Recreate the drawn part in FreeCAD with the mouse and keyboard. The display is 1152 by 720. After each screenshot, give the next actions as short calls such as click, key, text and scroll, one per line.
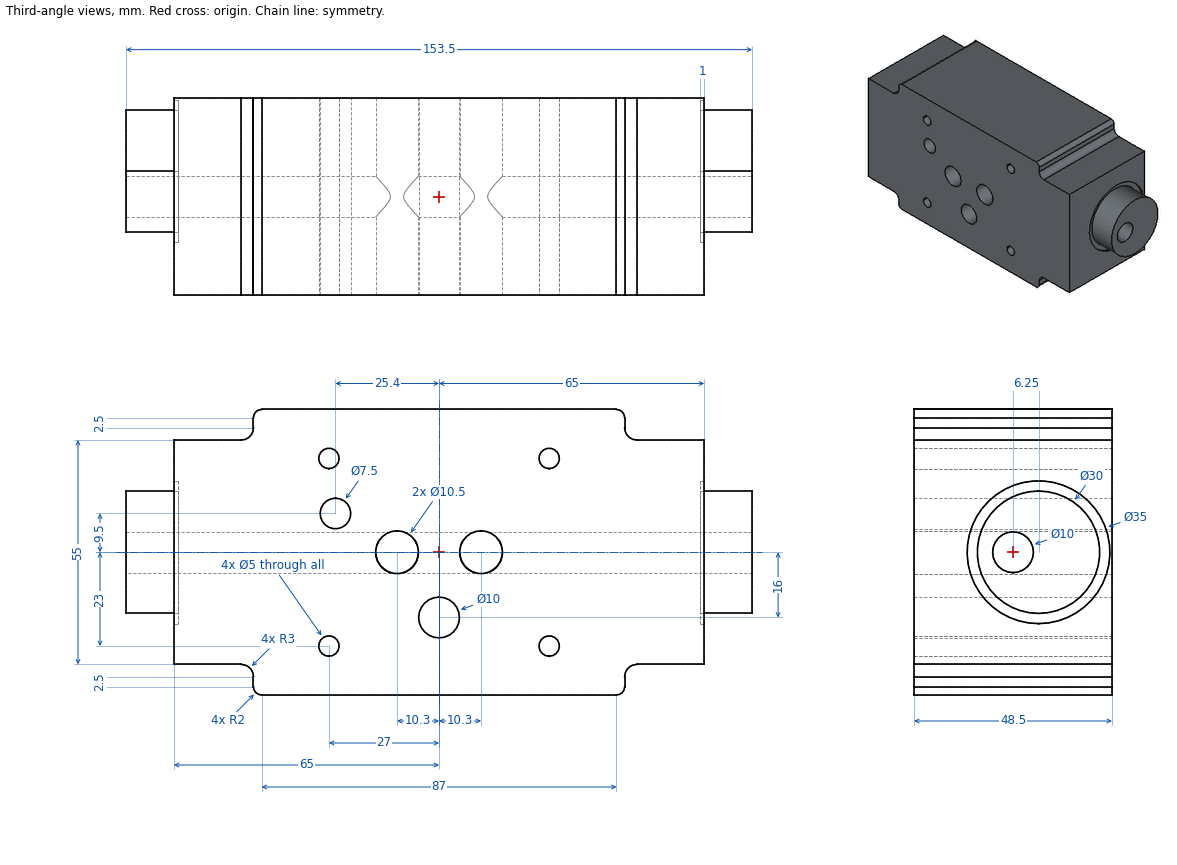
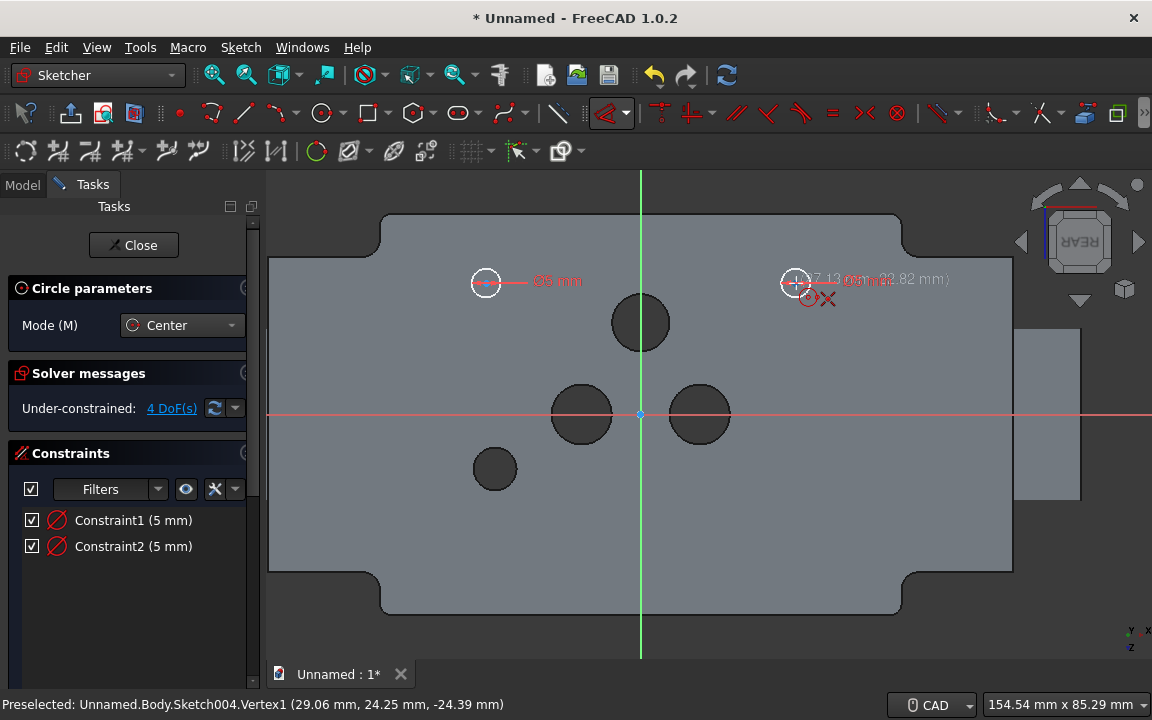
scroll(796, 546, up, 3)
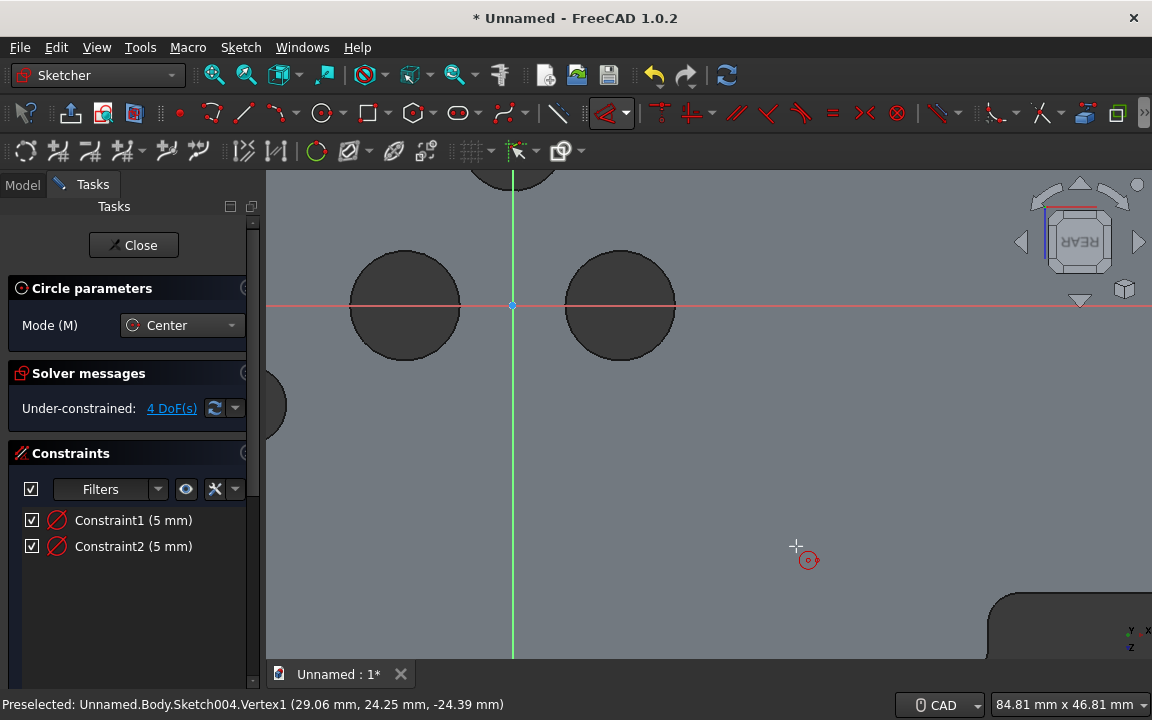
click(795, 546)
move(813, 528)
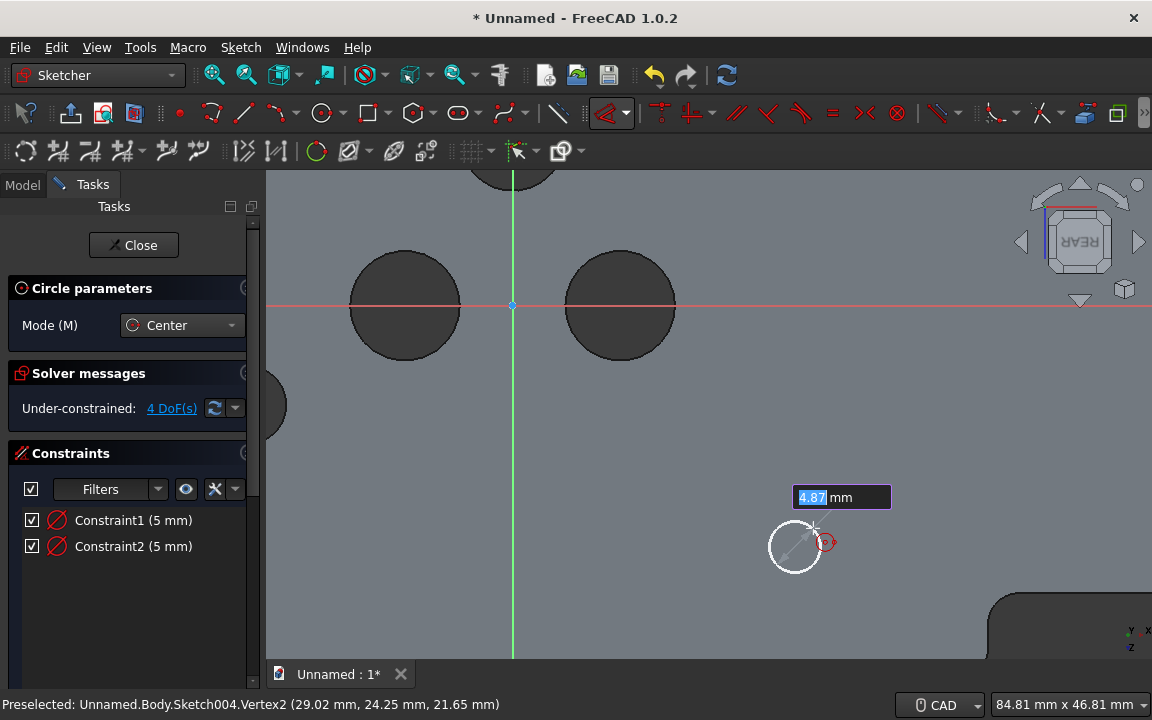
text(5)
key(Return)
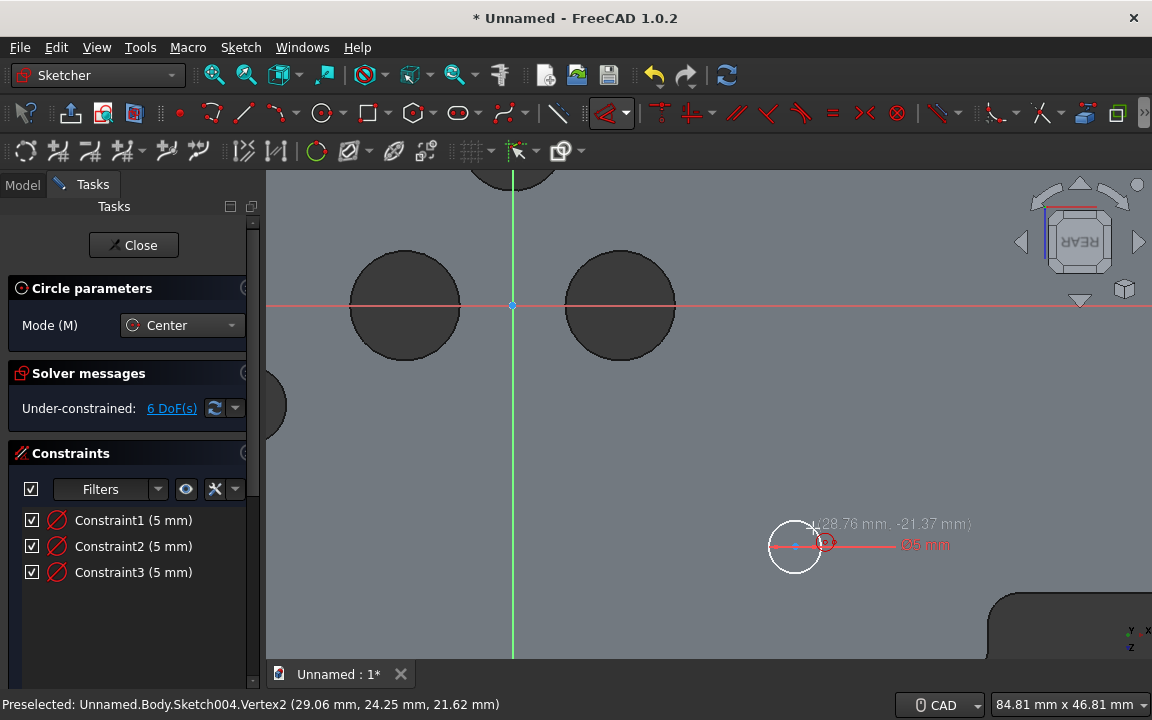
scroll(796, 547, down, 3)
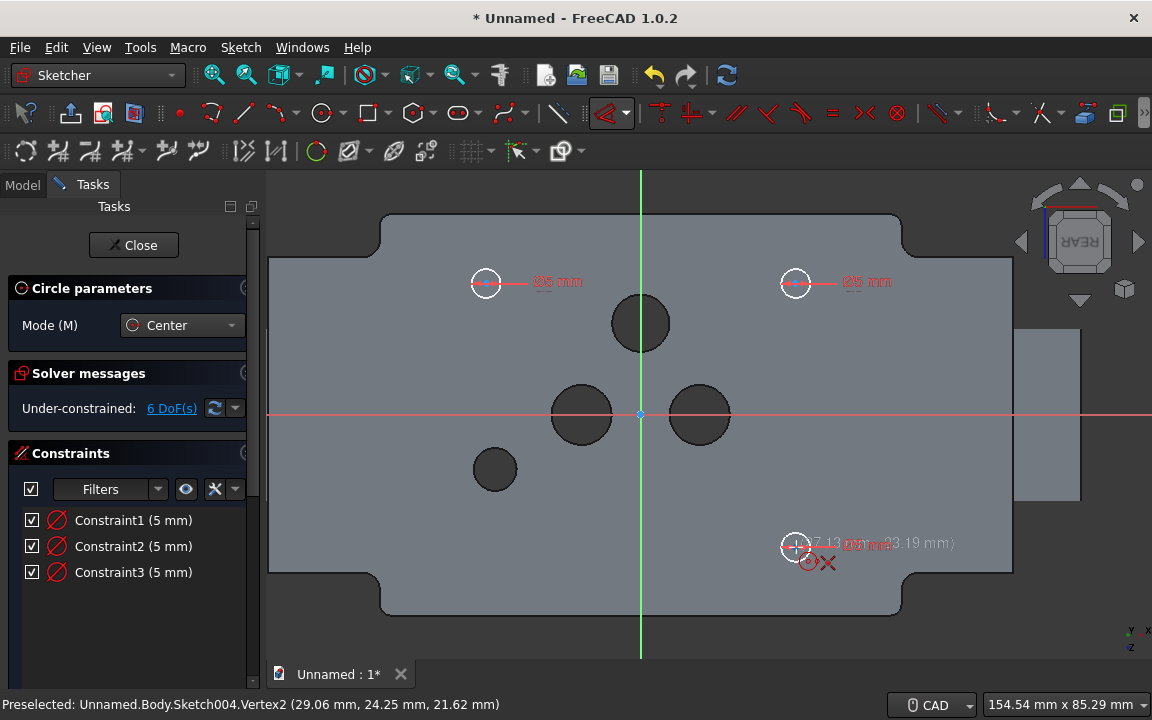
scroll(486, 547, up, 3)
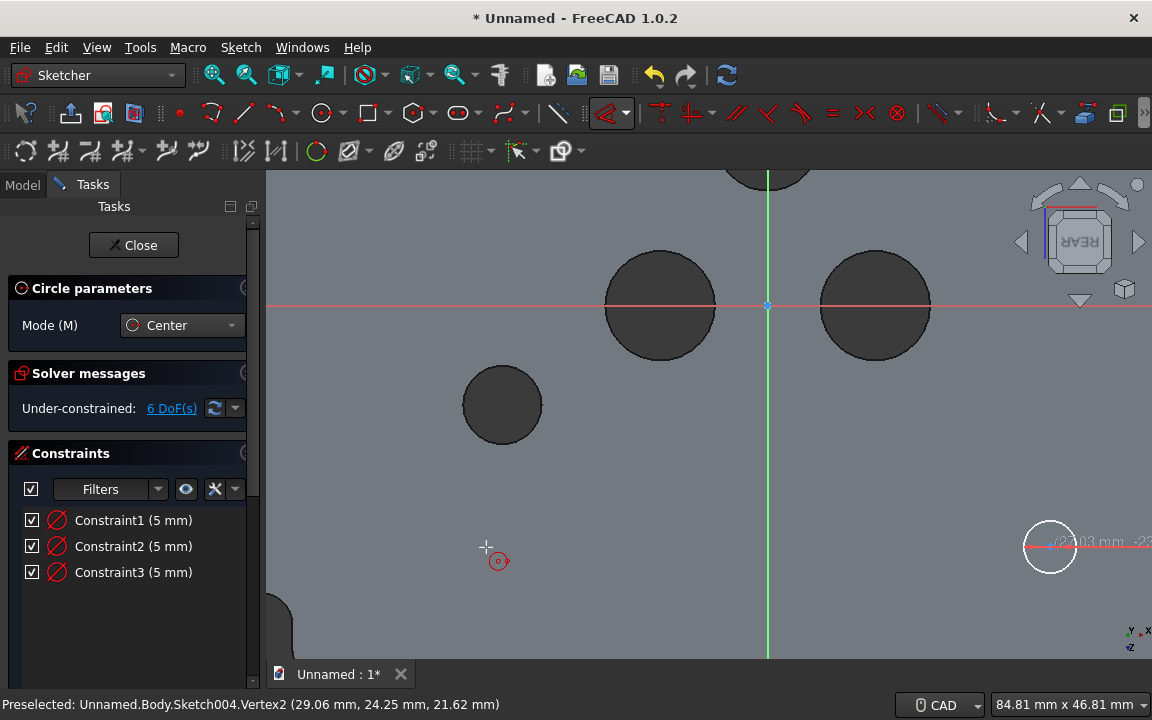
click(486, 546)
move(504, 528)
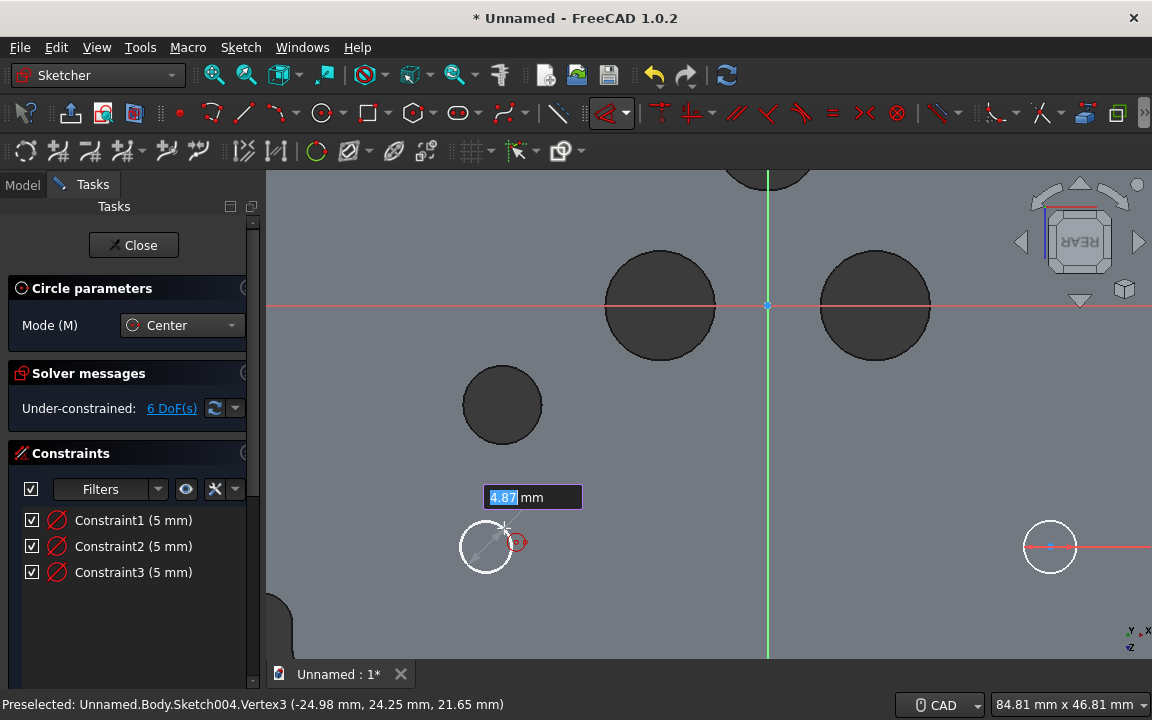
text(5)
key(Return)
key(Escape)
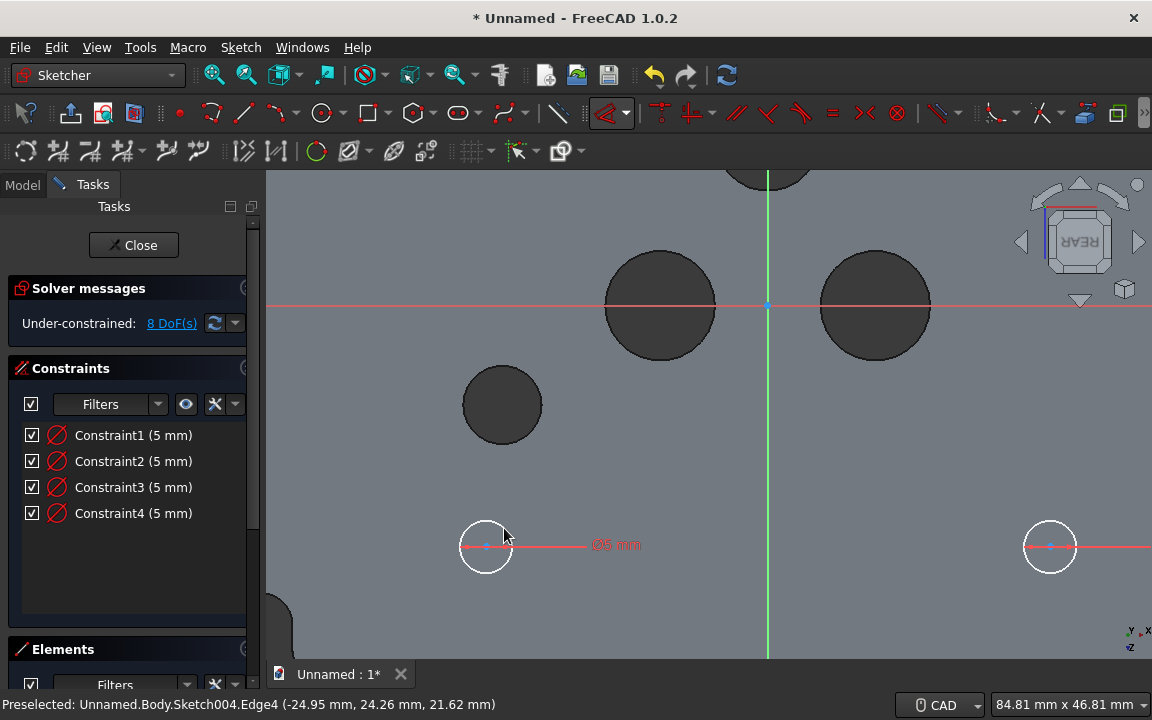
scroll(486, 547, down, 3)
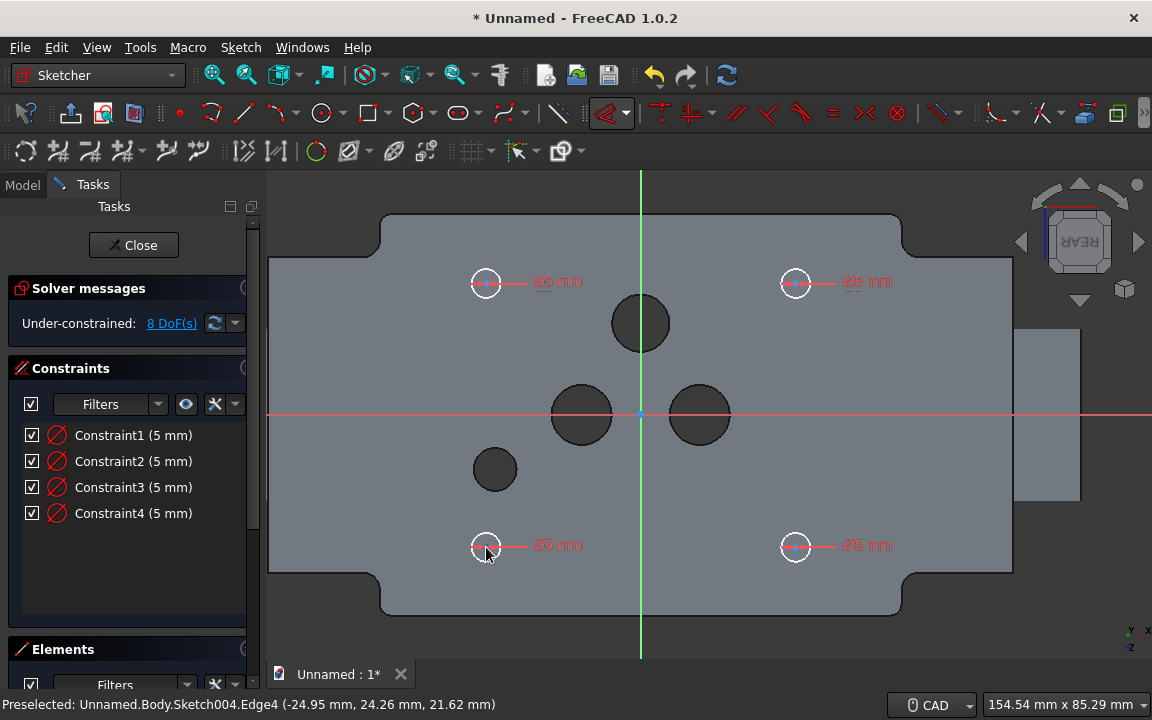
click(486, 284)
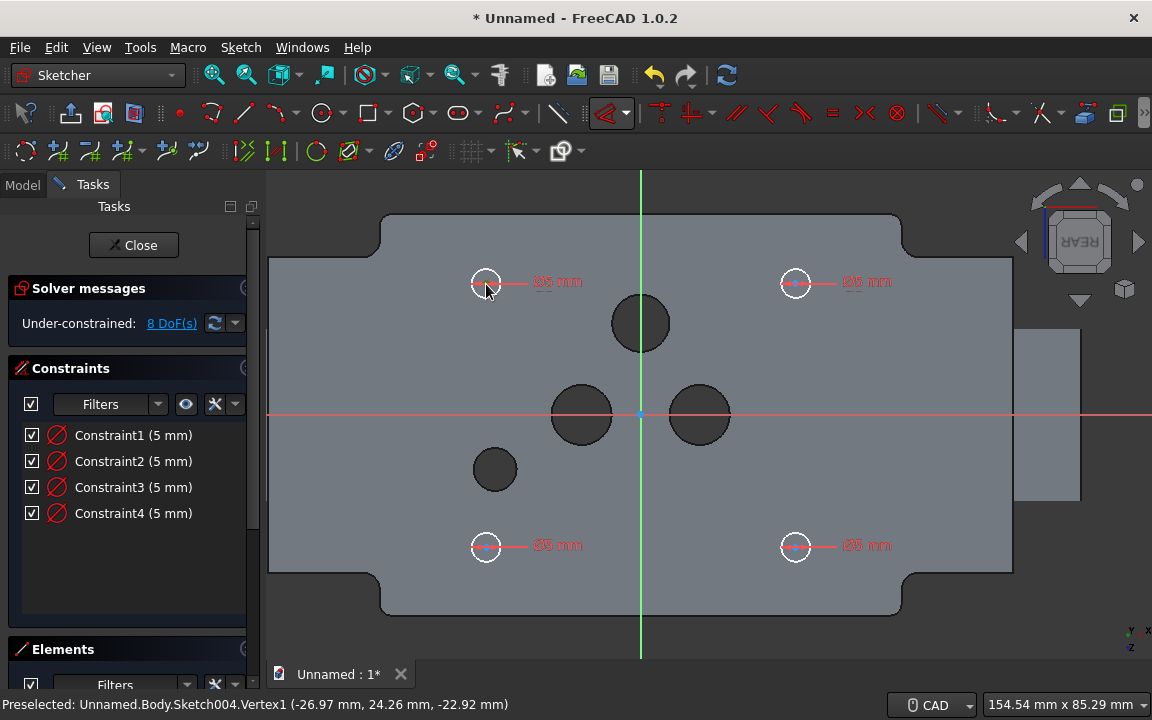
click(796, 284)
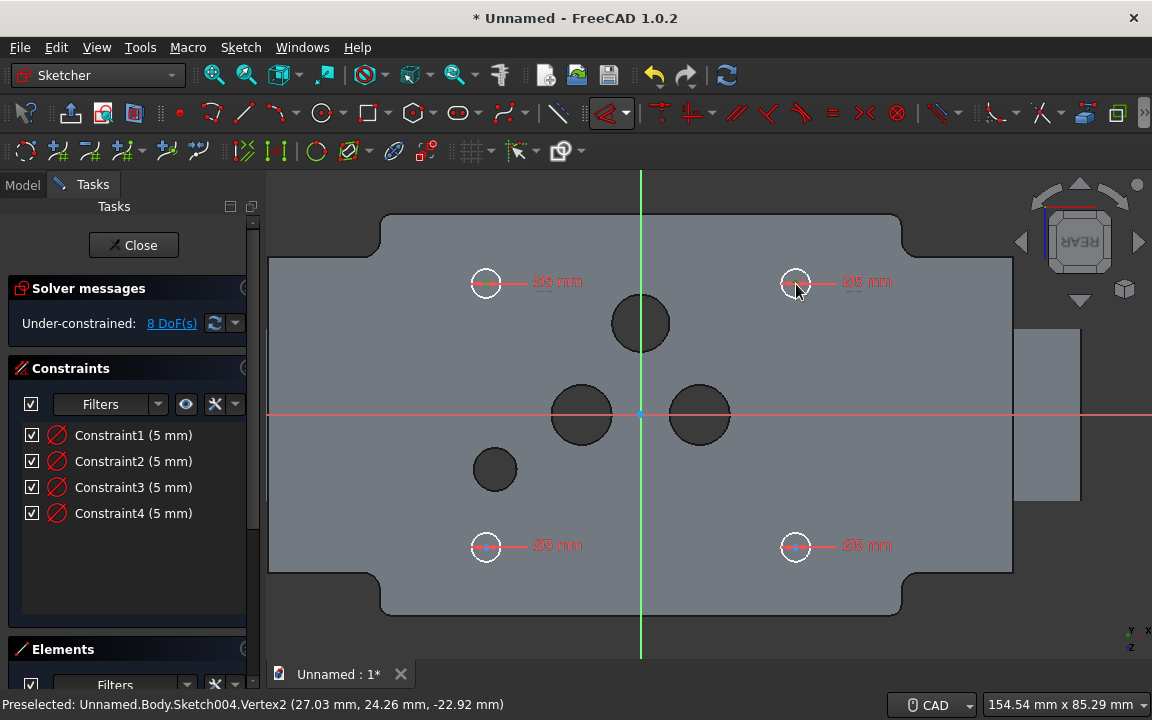
click(641, 600)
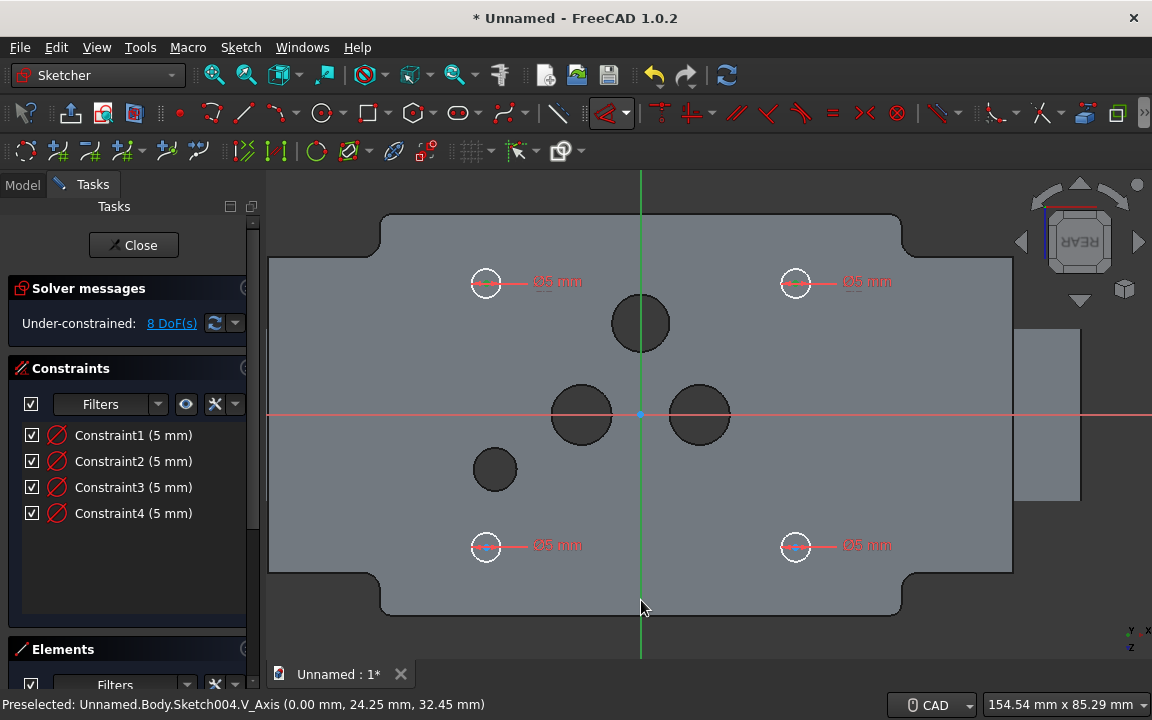
click(866, 114)